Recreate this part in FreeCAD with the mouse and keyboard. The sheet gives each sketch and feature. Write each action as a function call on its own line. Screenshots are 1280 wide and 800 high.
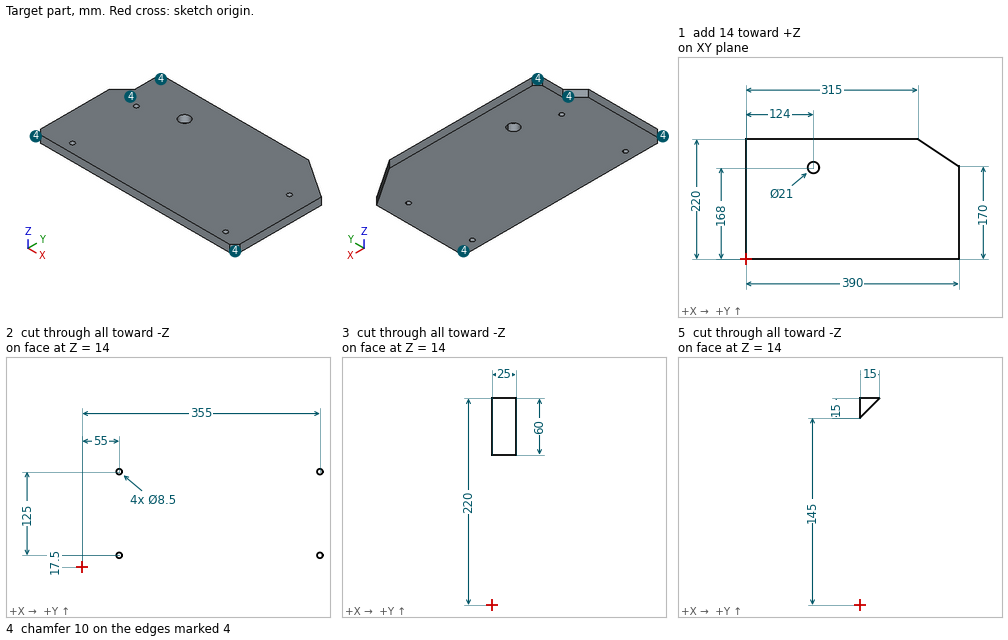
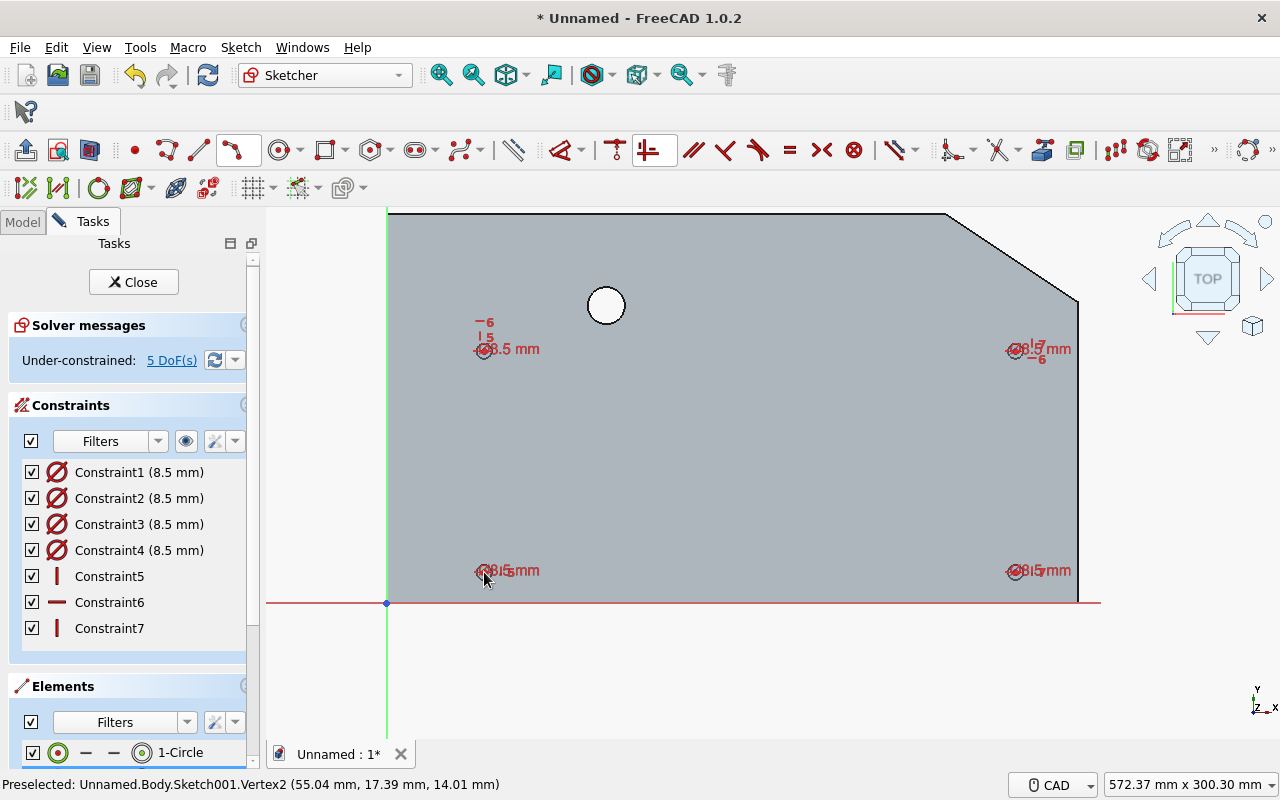
click(1016, 572)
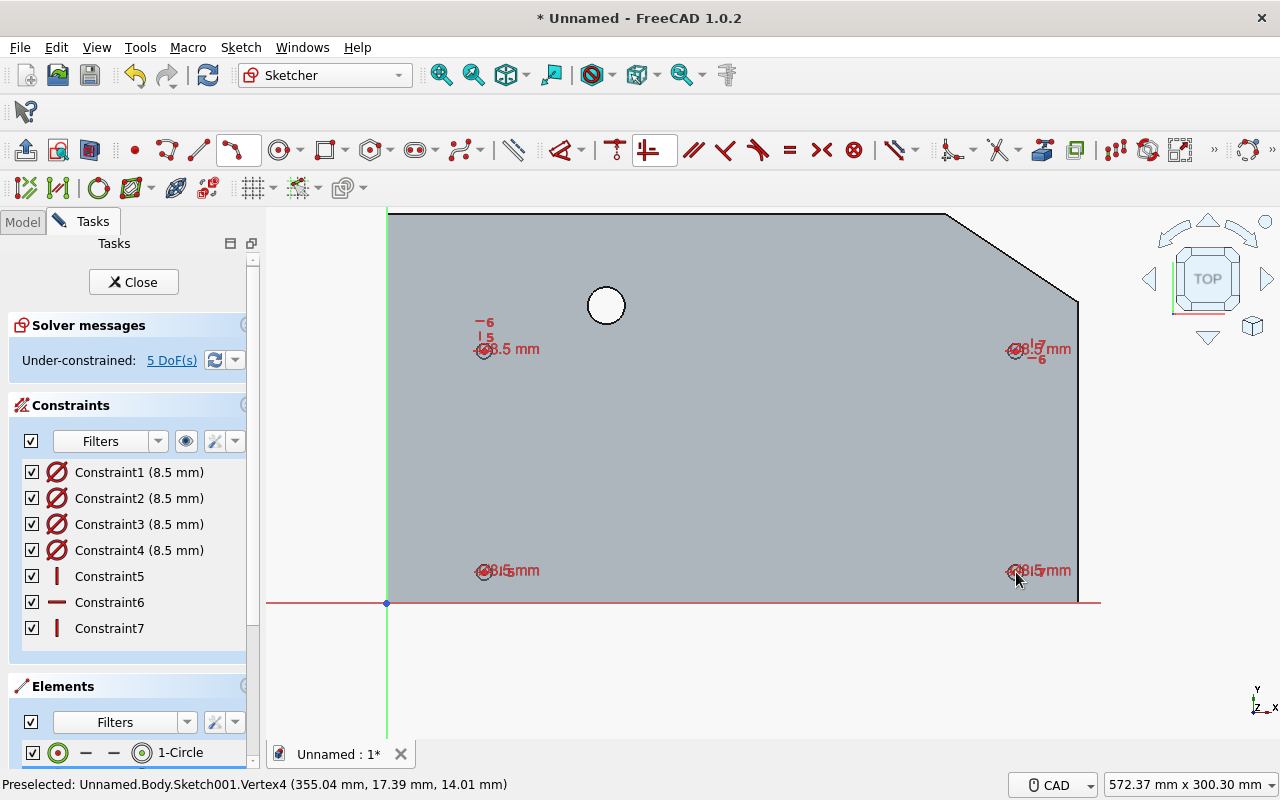
key(h)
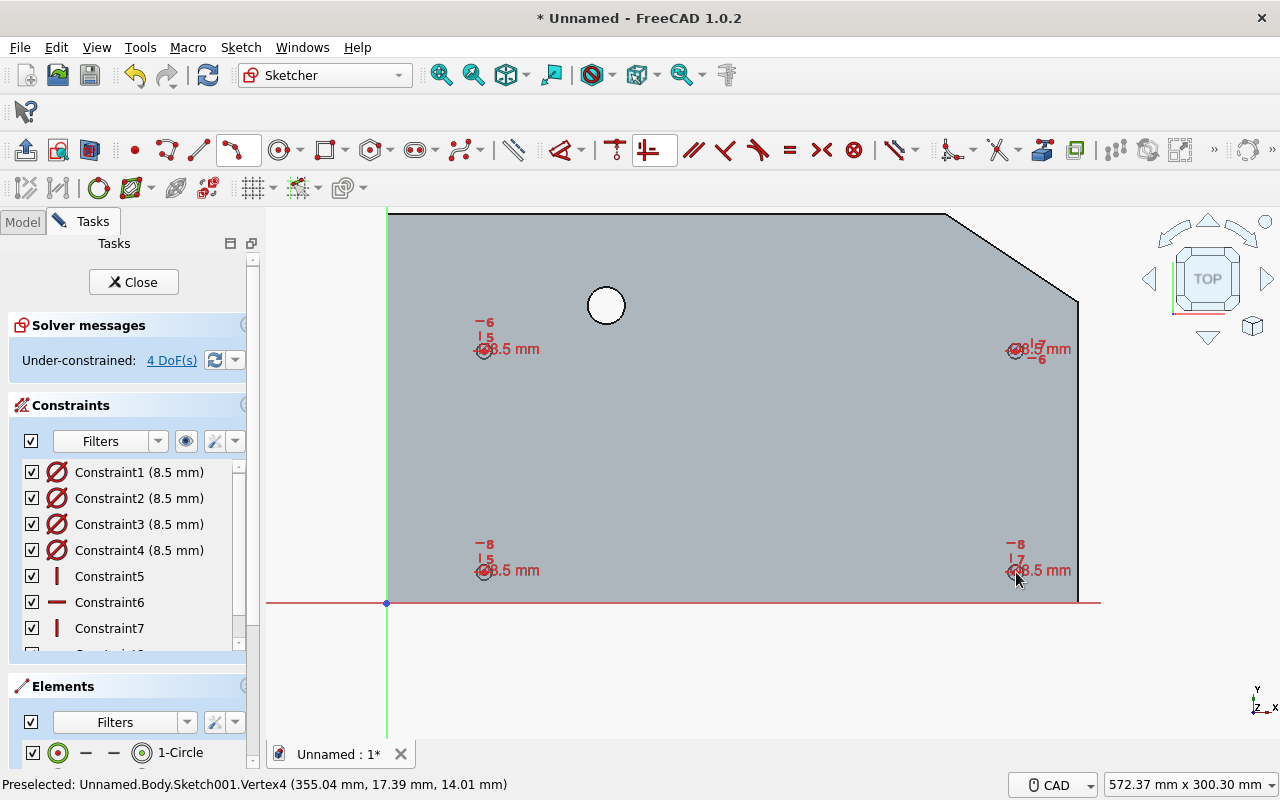
key(d)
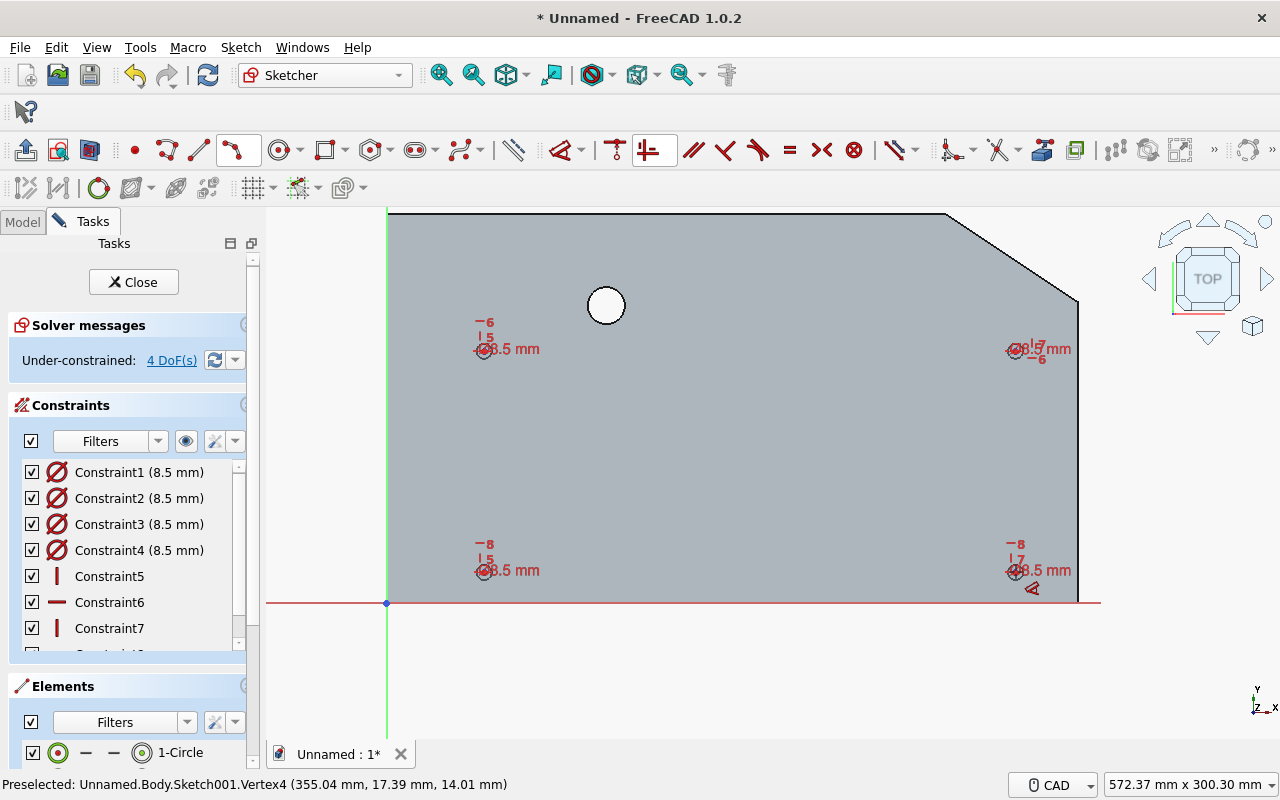
click(484, 351)
click(435, 637)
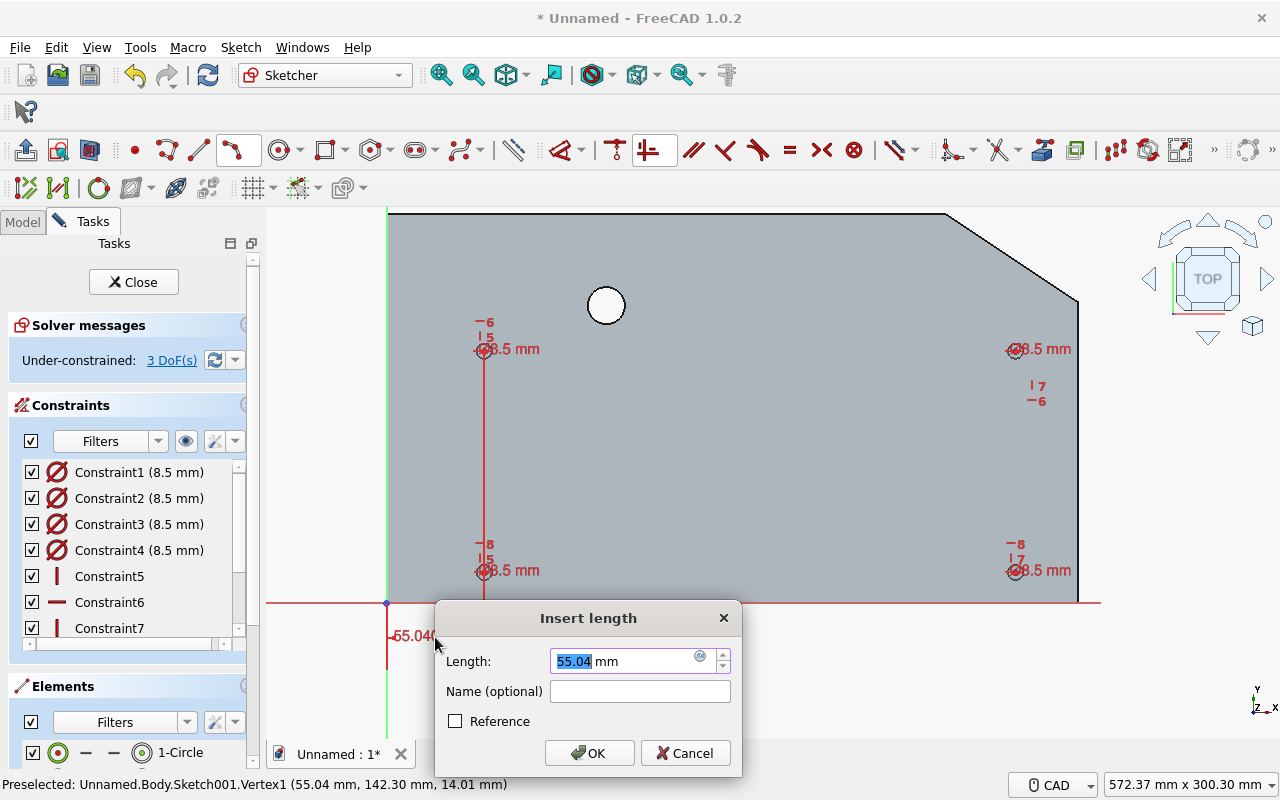
text(55)
key(Return)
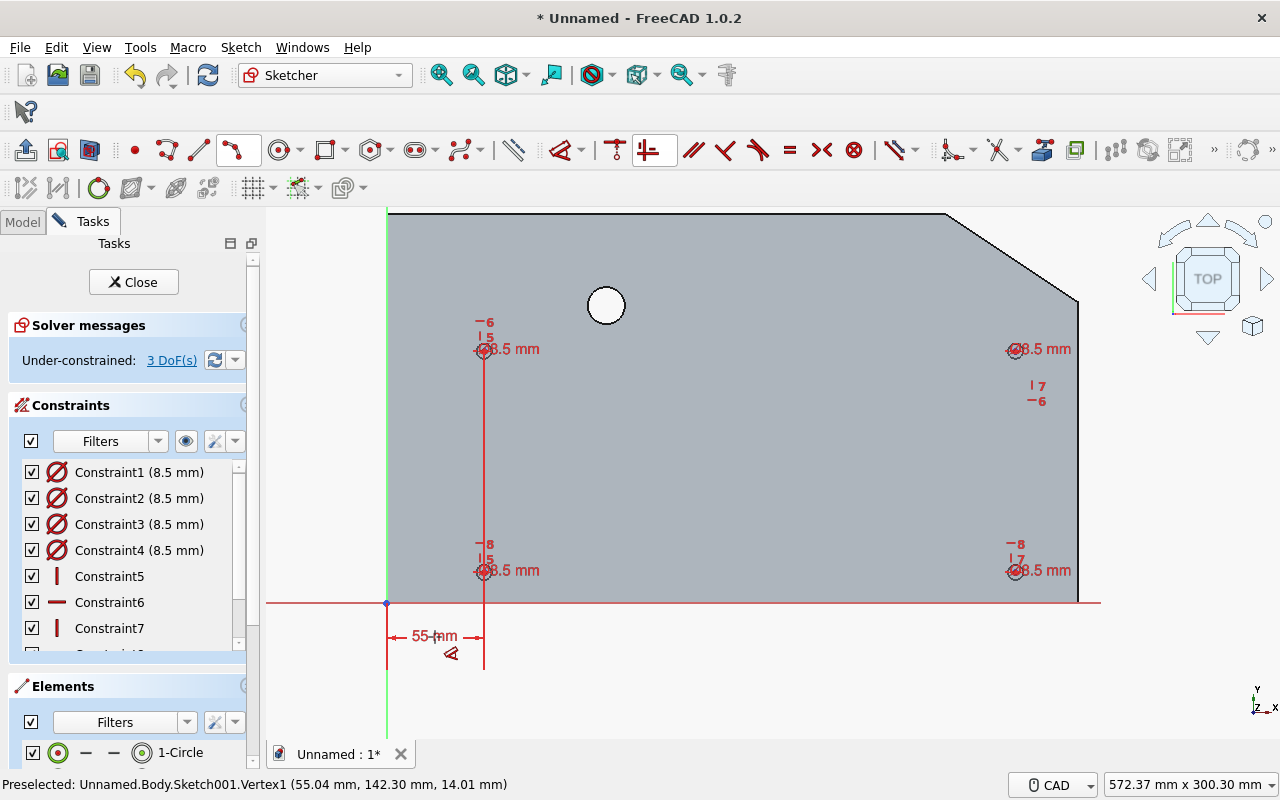
click(1016, 351)
click(701, 637)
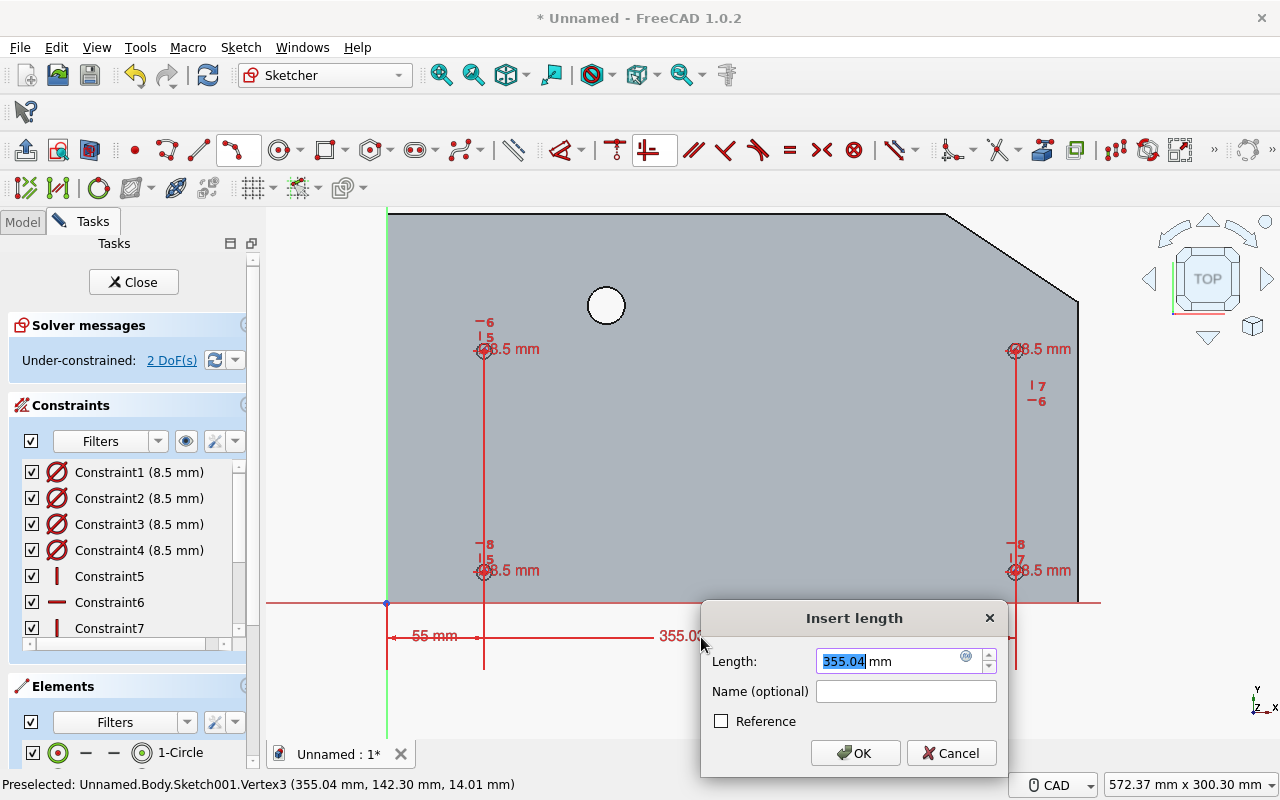
text(355)
key(Return)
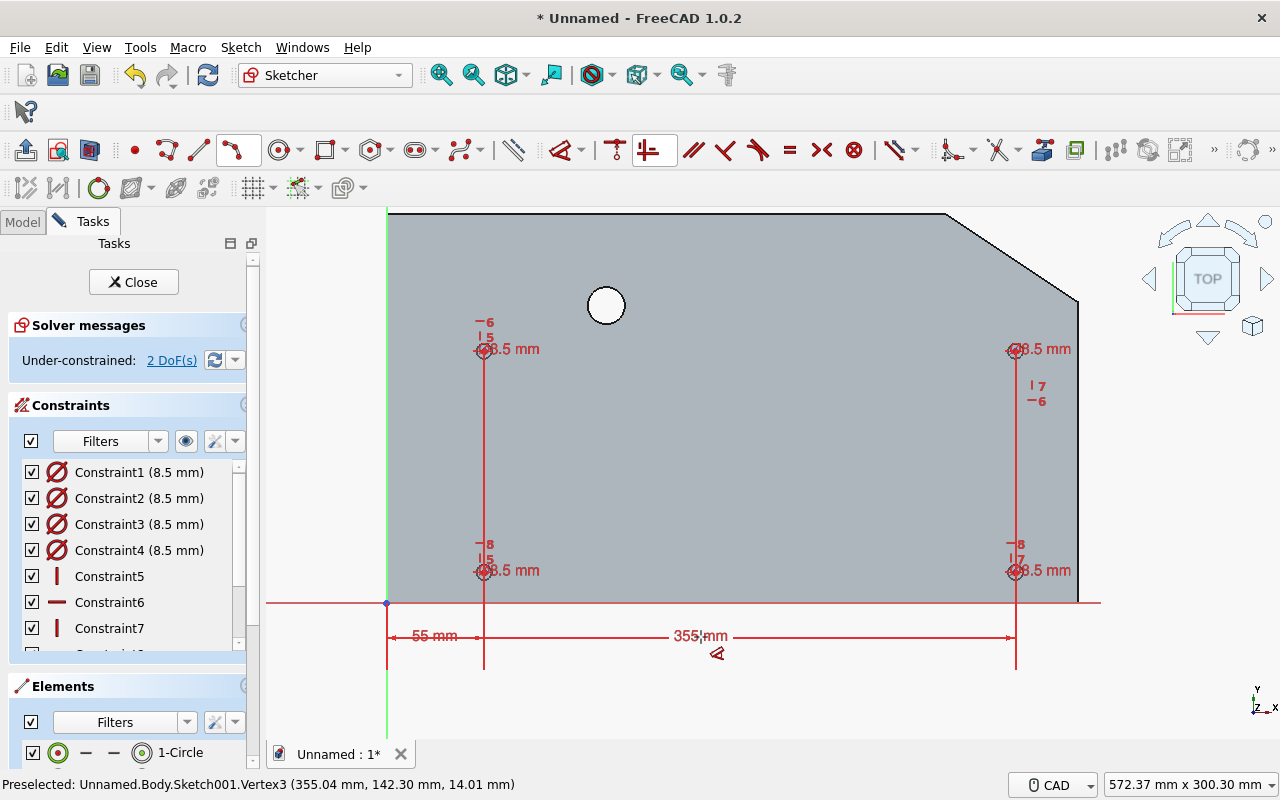
scroll(484, 572, up, 2)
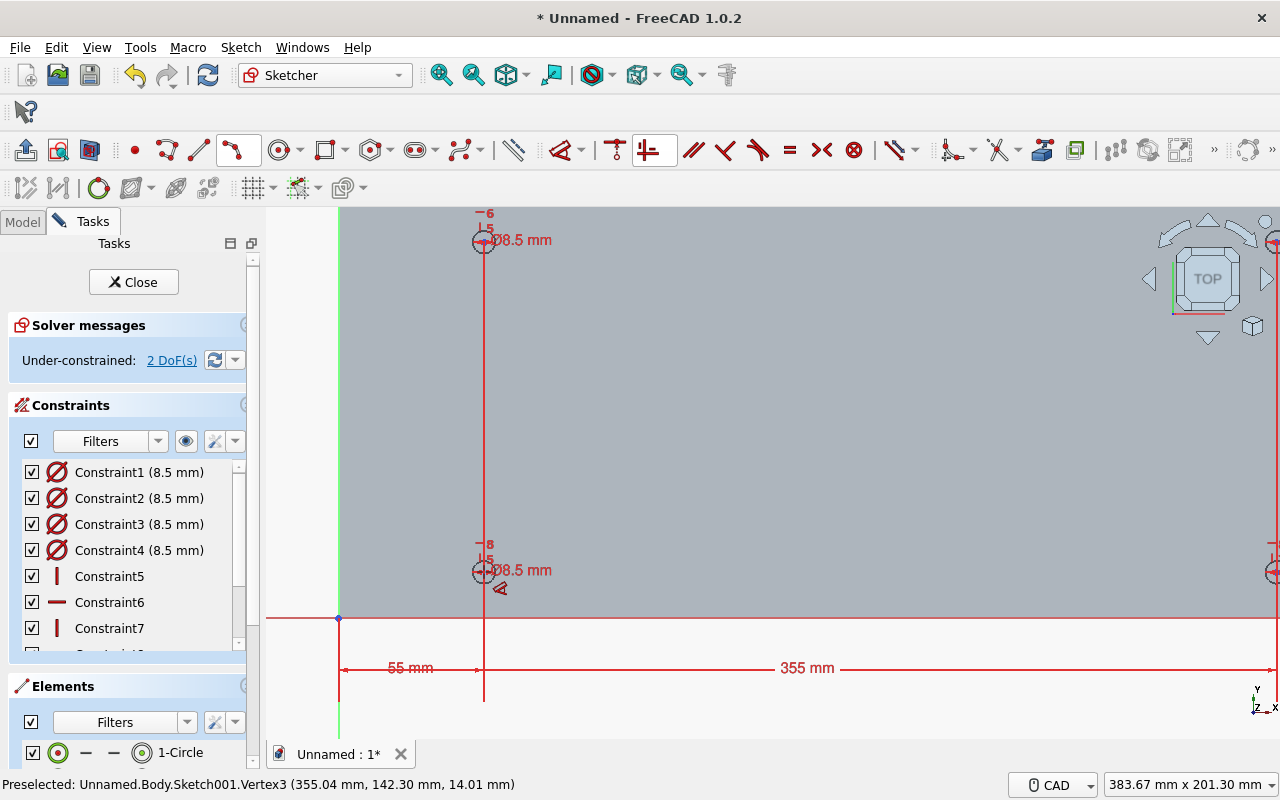
click(484, 572)
click(305, 595)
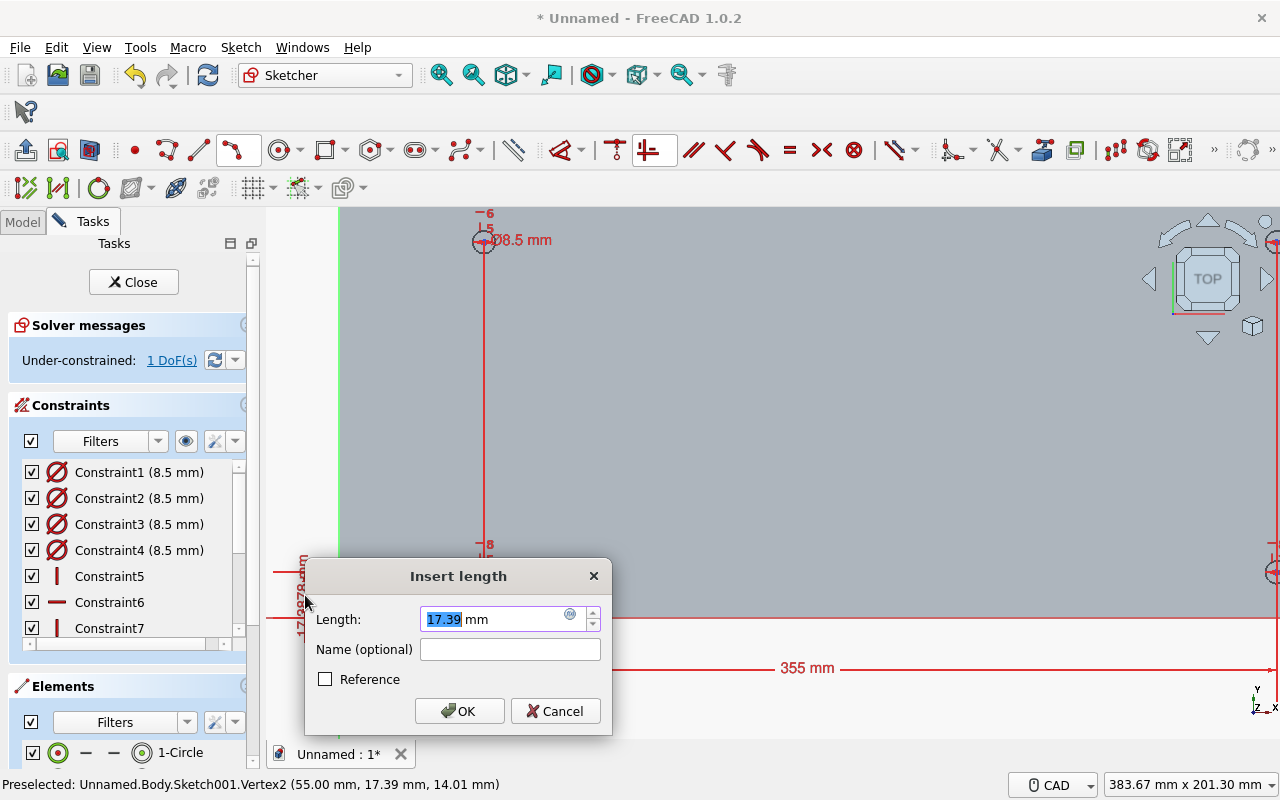
text(17.5)
key(Return)